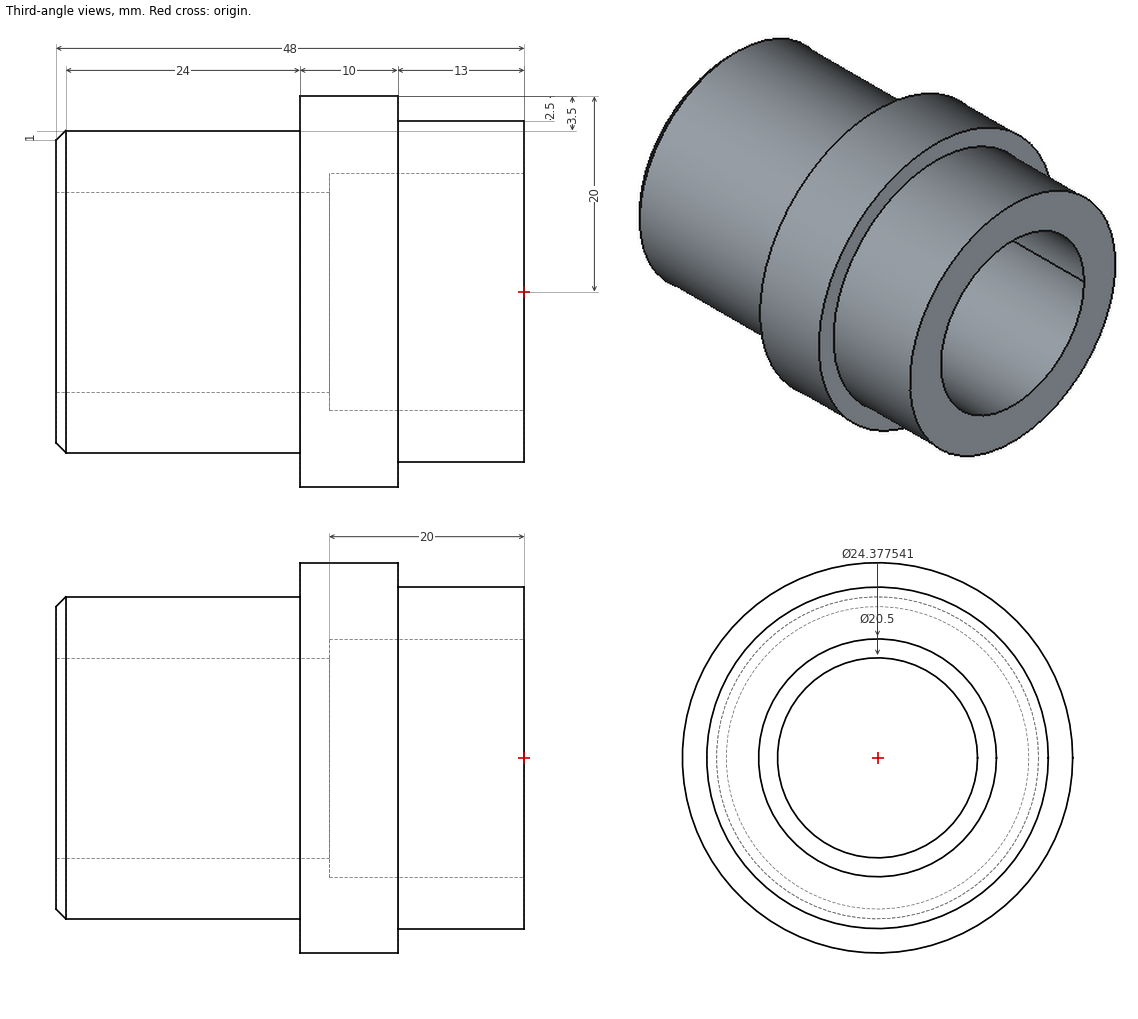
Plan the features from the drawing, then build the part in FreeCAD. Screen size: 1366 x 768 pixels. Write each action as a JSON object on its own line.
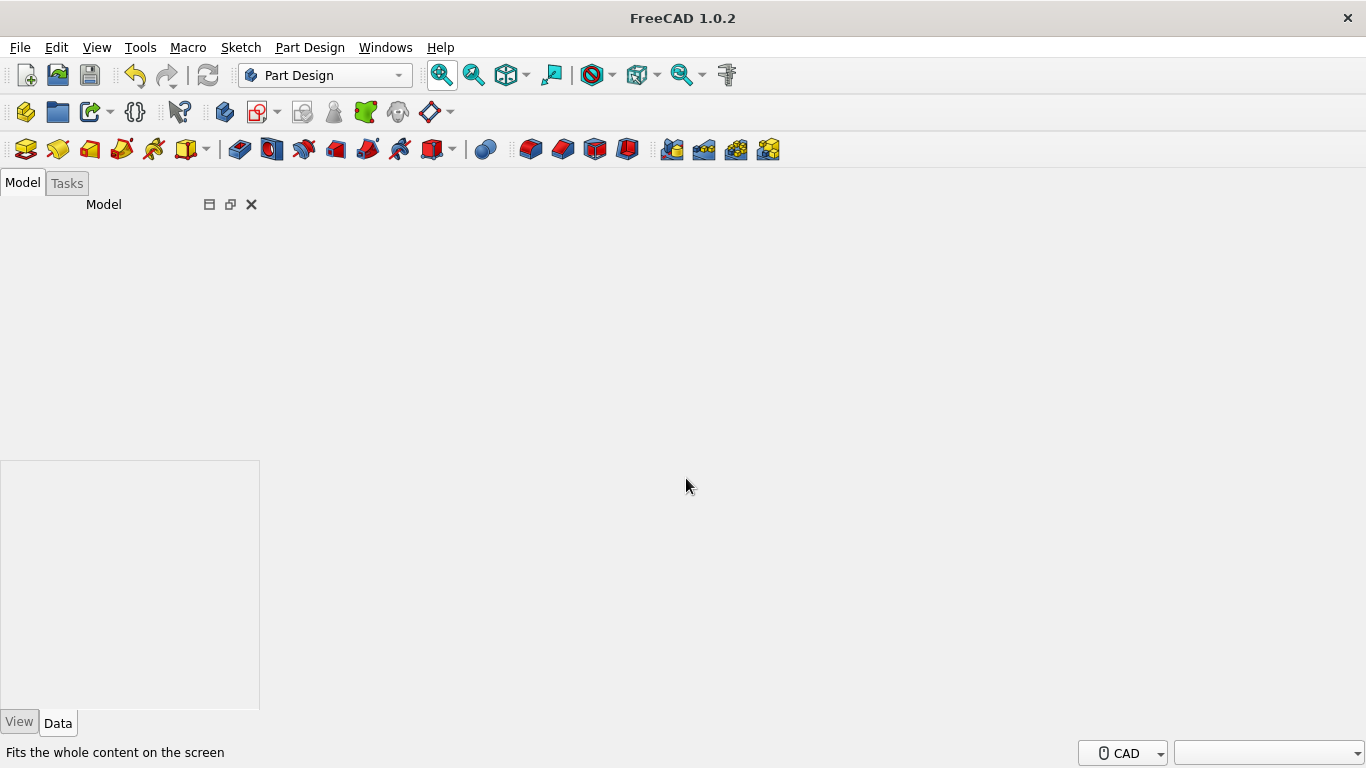
{"action": "left_click", "coordinate": [26, 76]}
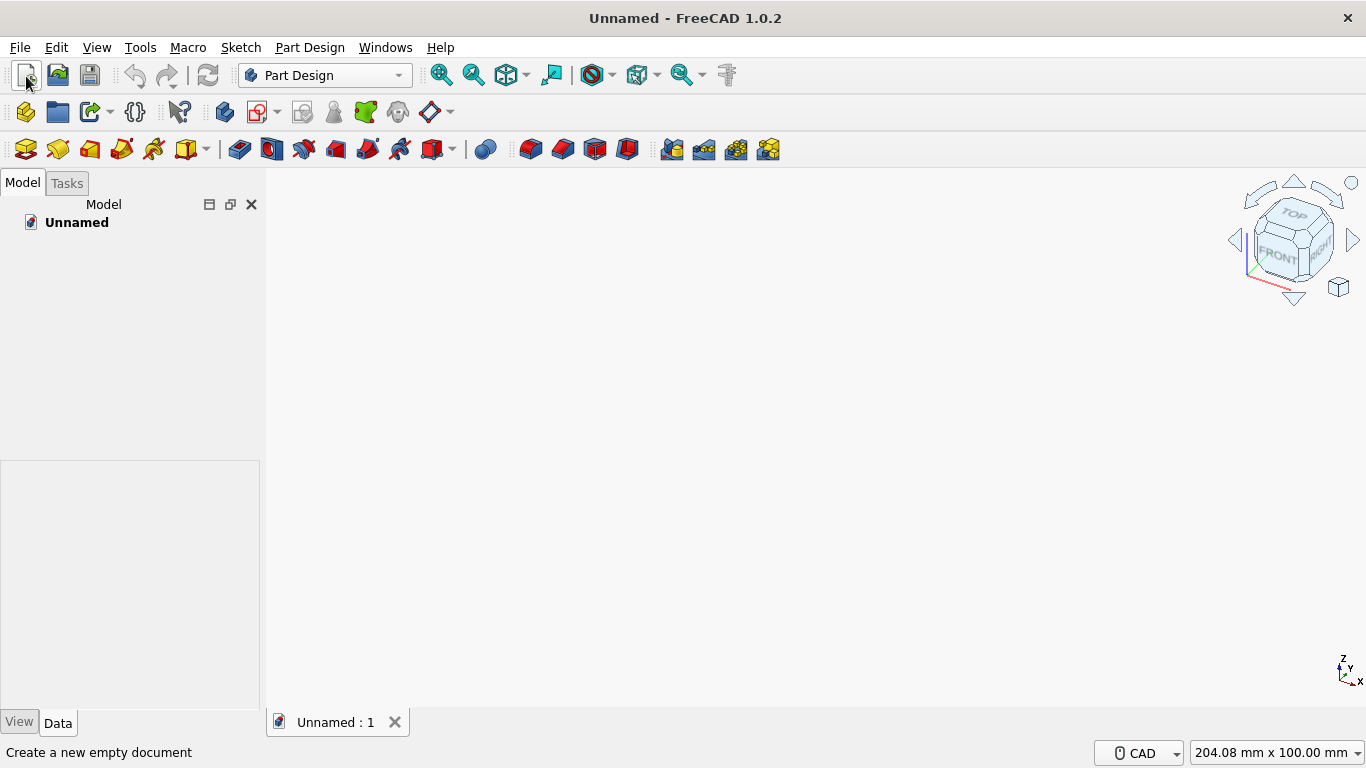
{"action": "left_click", "coordinate": [258, 112]}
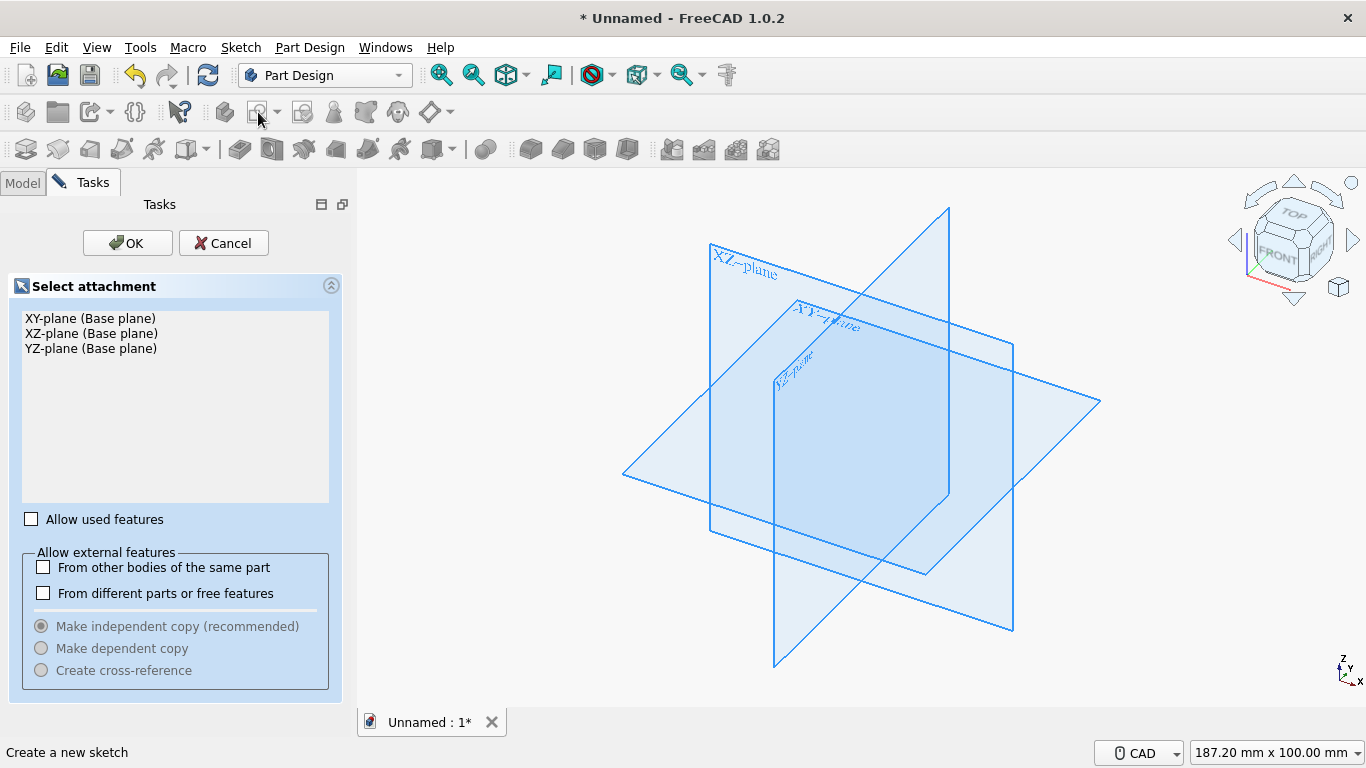
{"action": "left_click", "coordinate": [82, 318]}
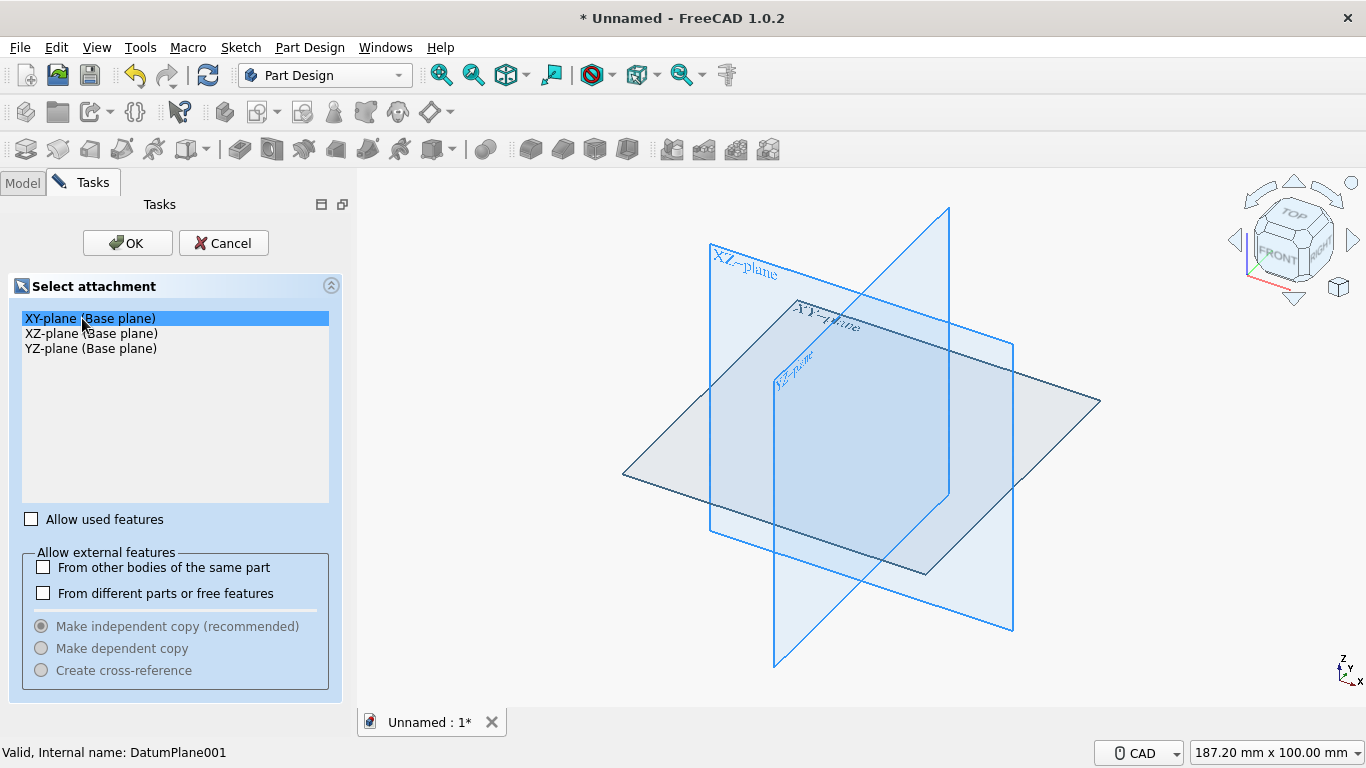
{"action": "left_click", "coordinate": [128, 243]}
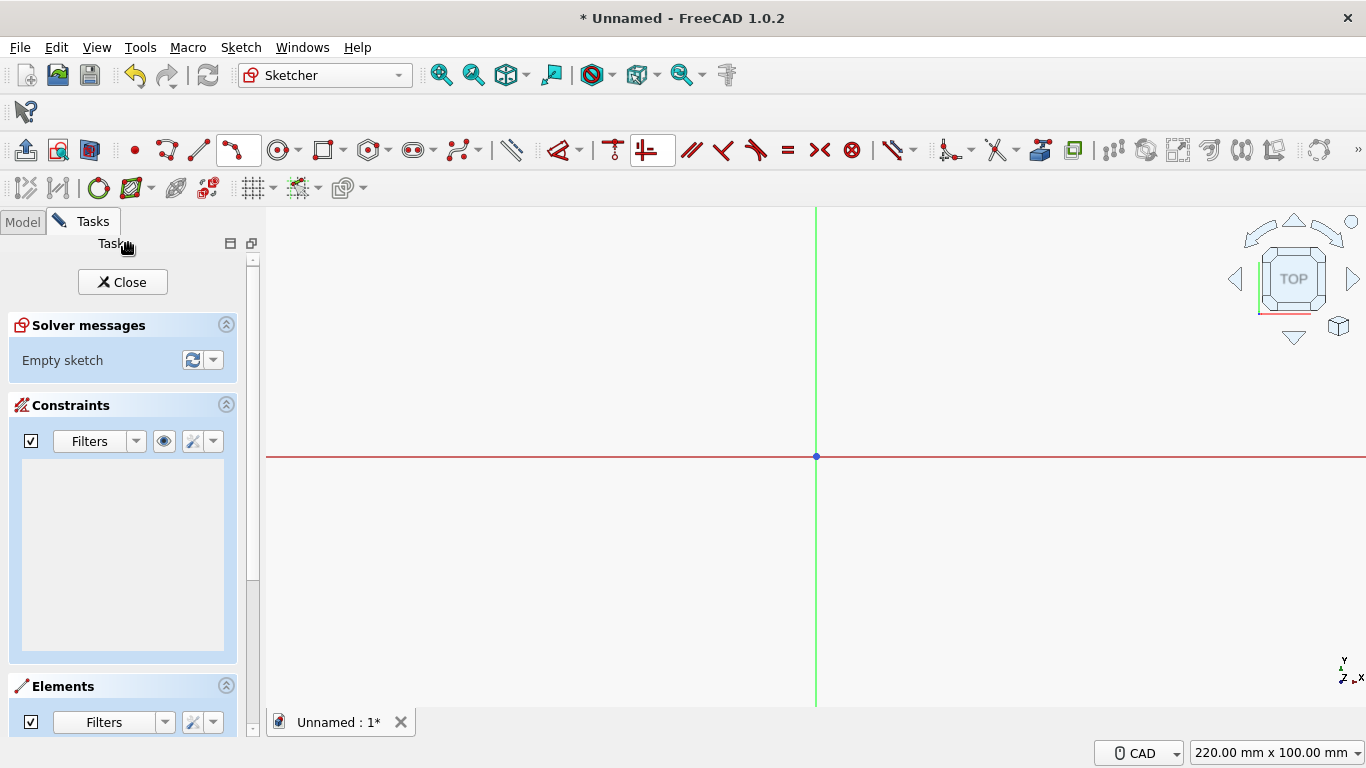
{"action": "scroll", "coordinate": [666, 378], "scroll_direction": "up", "scroll_amount": 5}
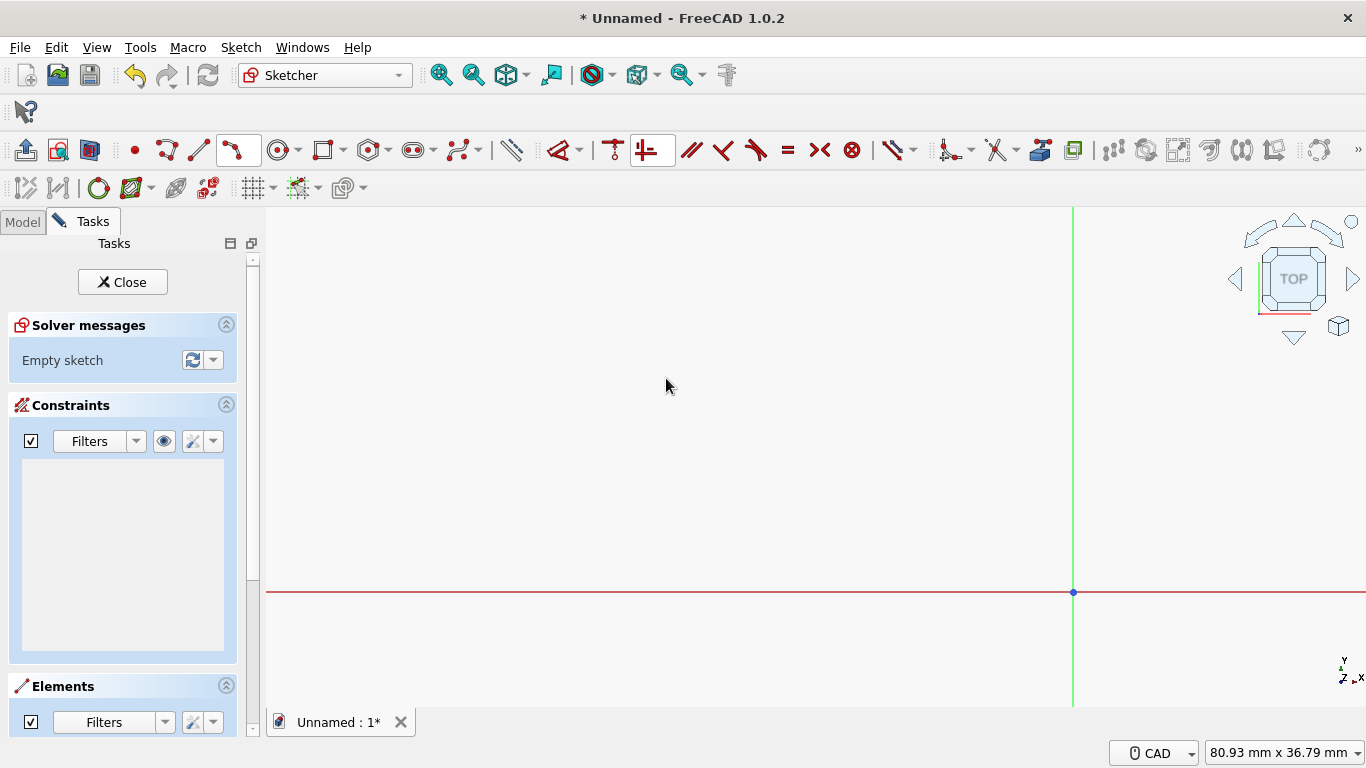
{"action": "key", "text": "g m"}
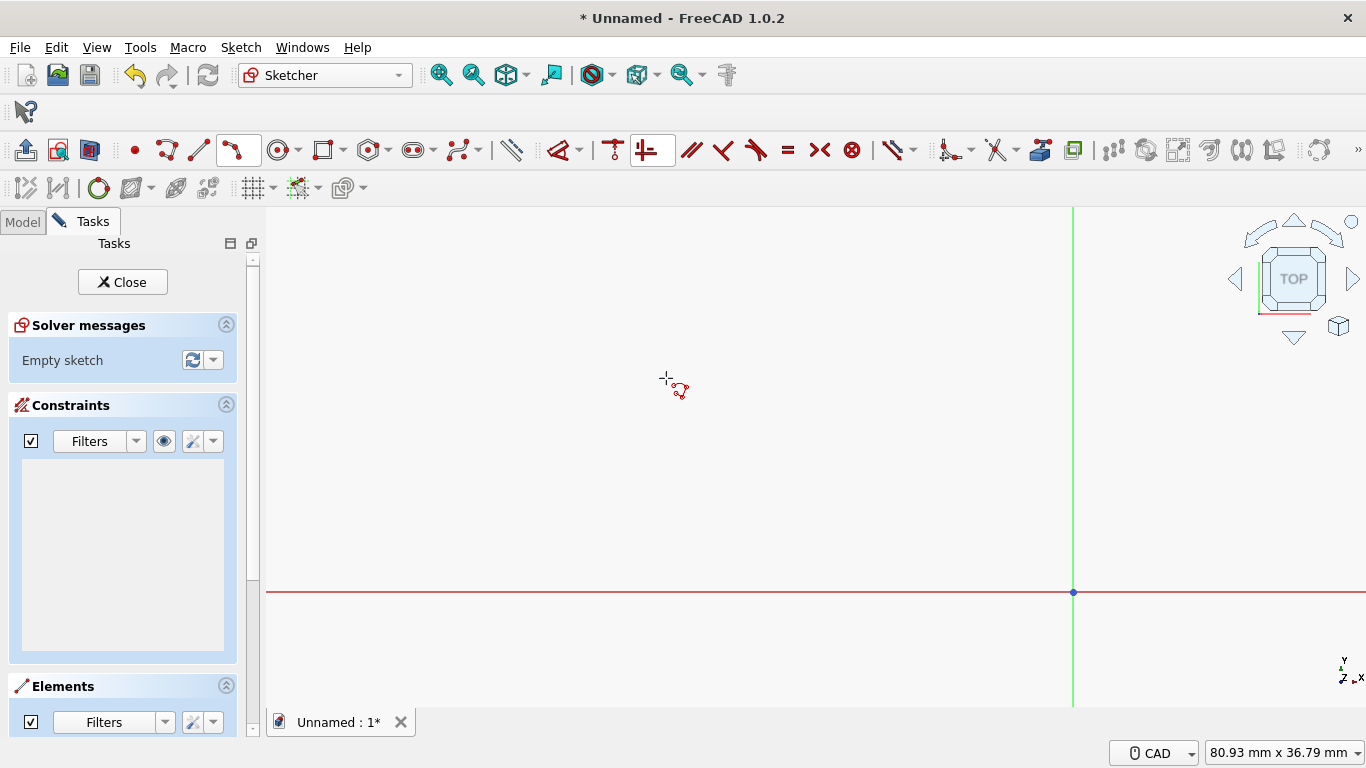
{"action": "left_click", "coordinate": [1073, 592]}
{"action": "left_click", "coordinate": [1064, 354]}
{"action": "left_click", "coordinate": [896, 354]}
{"action": "left_click", "coordinate": [896, 320]}
{"action": "left_click", "coordinate": [761, 320]}
{"action": "left_click", "coordinate": [761, 368]}
{"action": "left_click", "coordinate": [434, 368]}
{"action": "left_click", "coordinate": [421, 381]}
{"action": "left_click", "coordinate": [421, 583]}
{"action": "left_click", "coordinate": [1073, 592]}
{"action": "key", "text": "Escape"}
{"action": "key", "text": "Escape"}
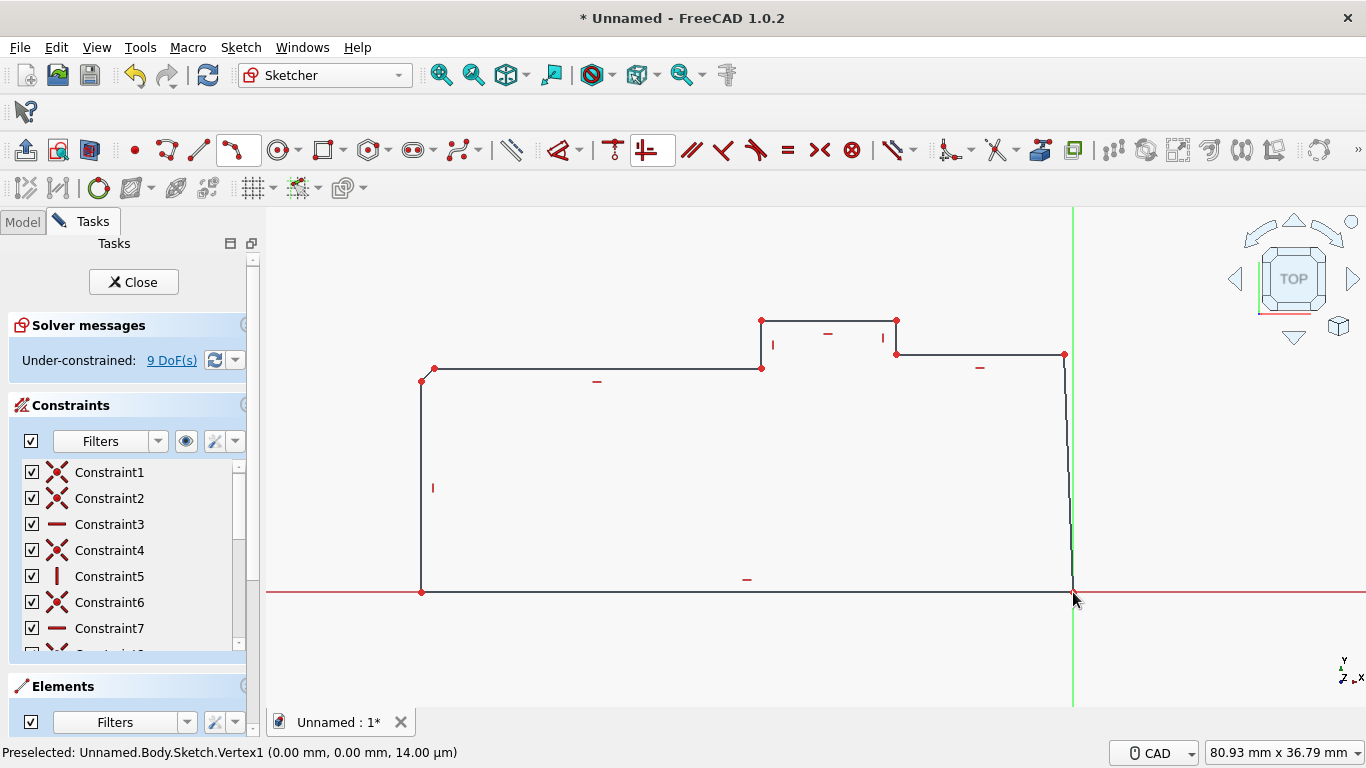
{"action": "left_click", "coordinate": [1070, 521]}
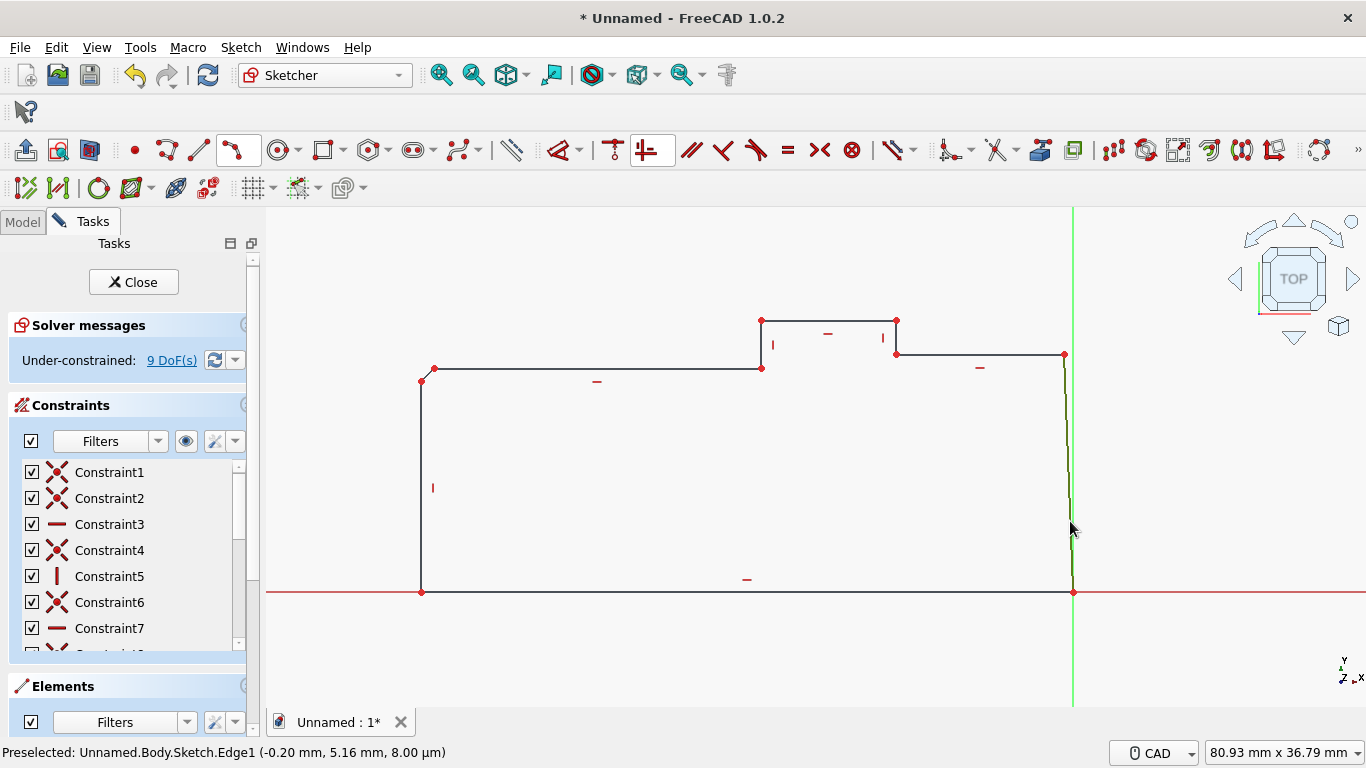
{"action": "key", "text": "v"}